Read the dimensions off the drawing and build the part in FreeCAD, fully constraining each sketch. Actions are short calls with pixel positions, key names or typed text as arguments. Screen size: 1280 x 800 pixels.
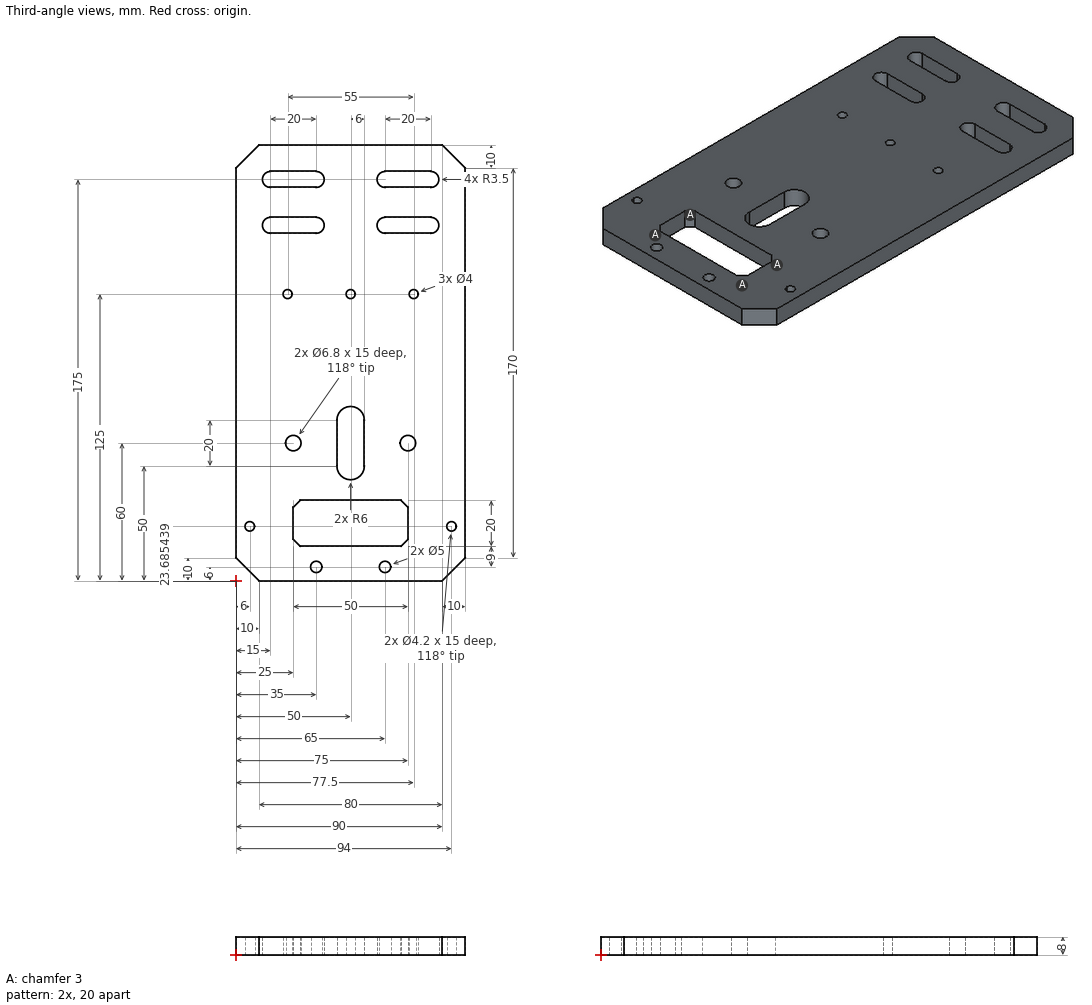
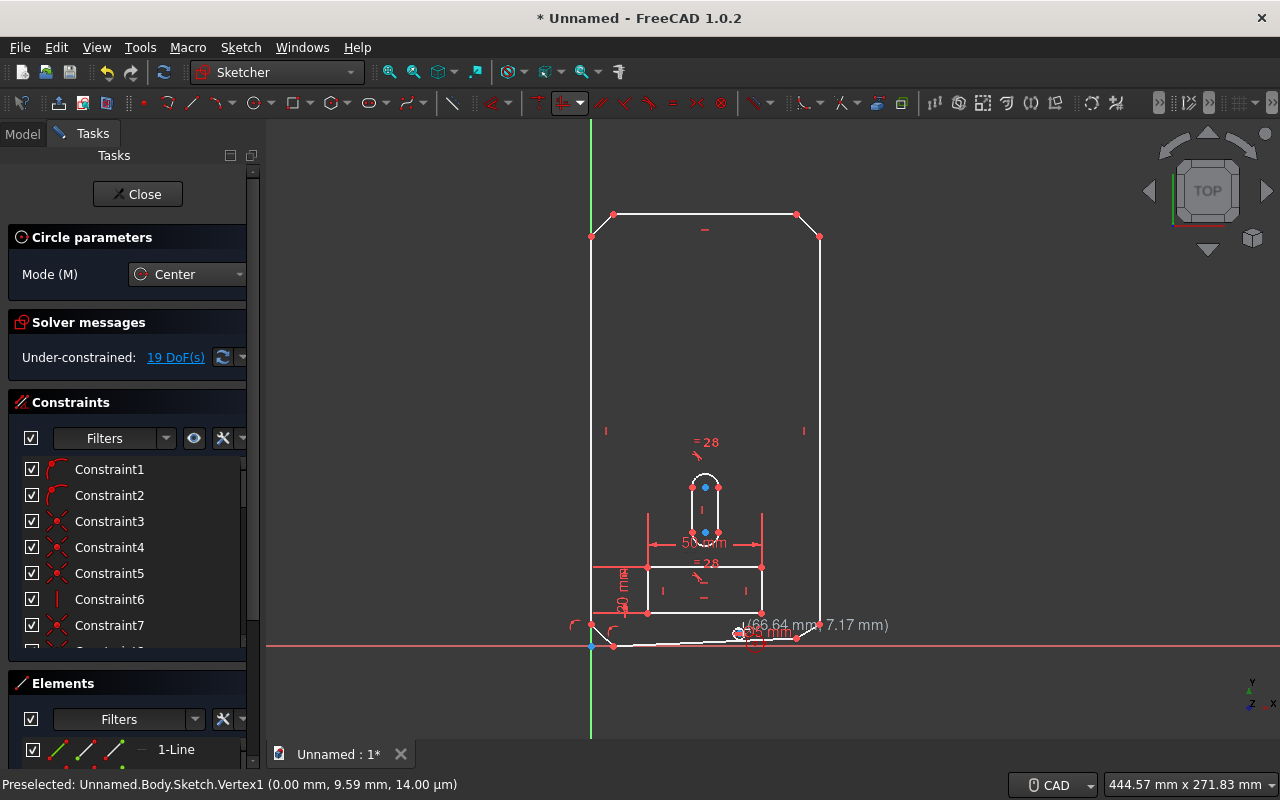
scroll(671, 633, up, 7)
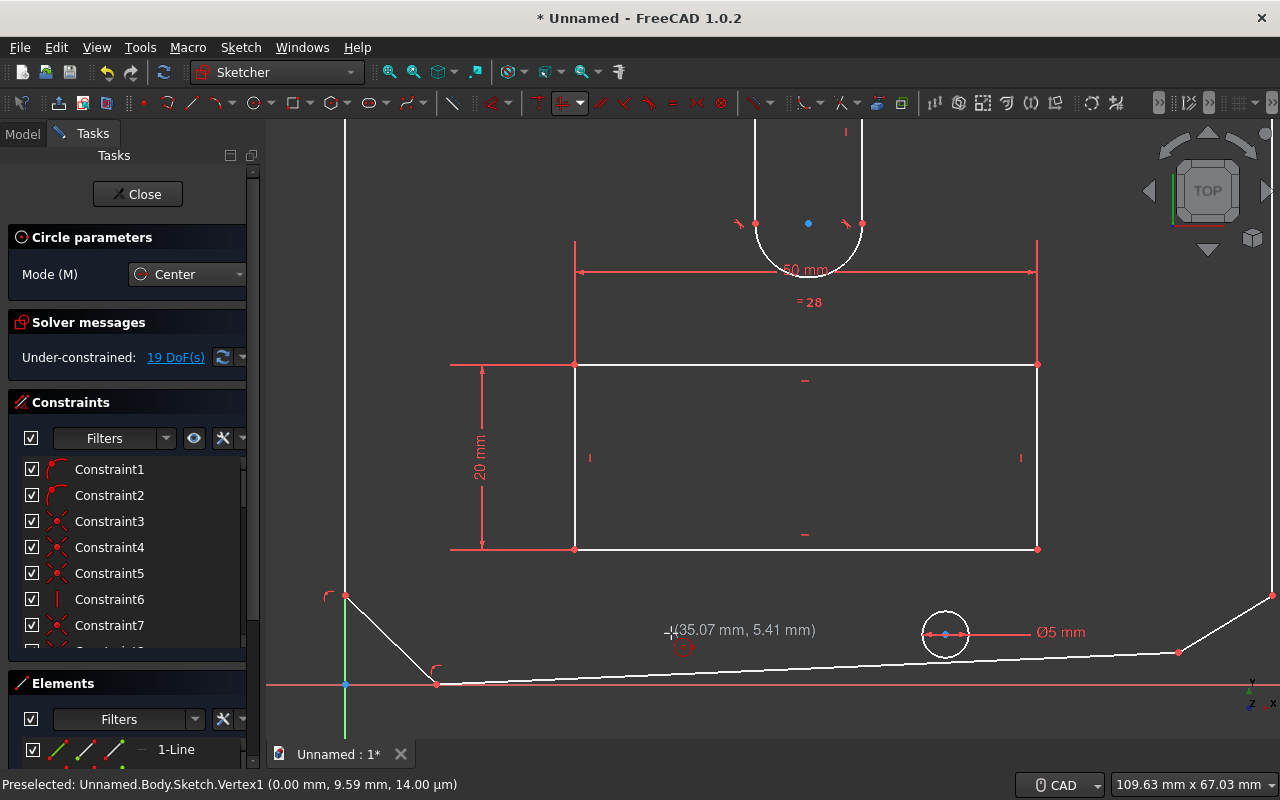
scroll(671, 633, down, 7)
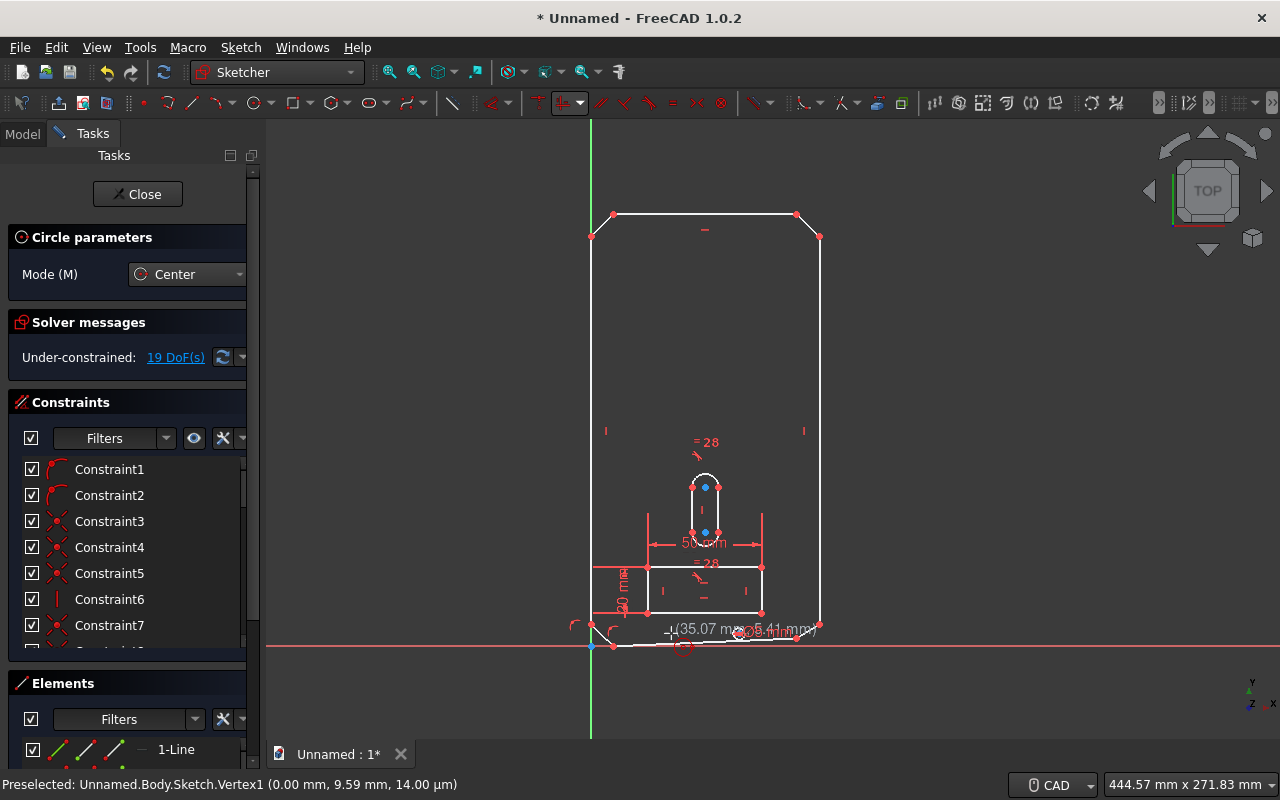
click(671, 633)
move(675, 629)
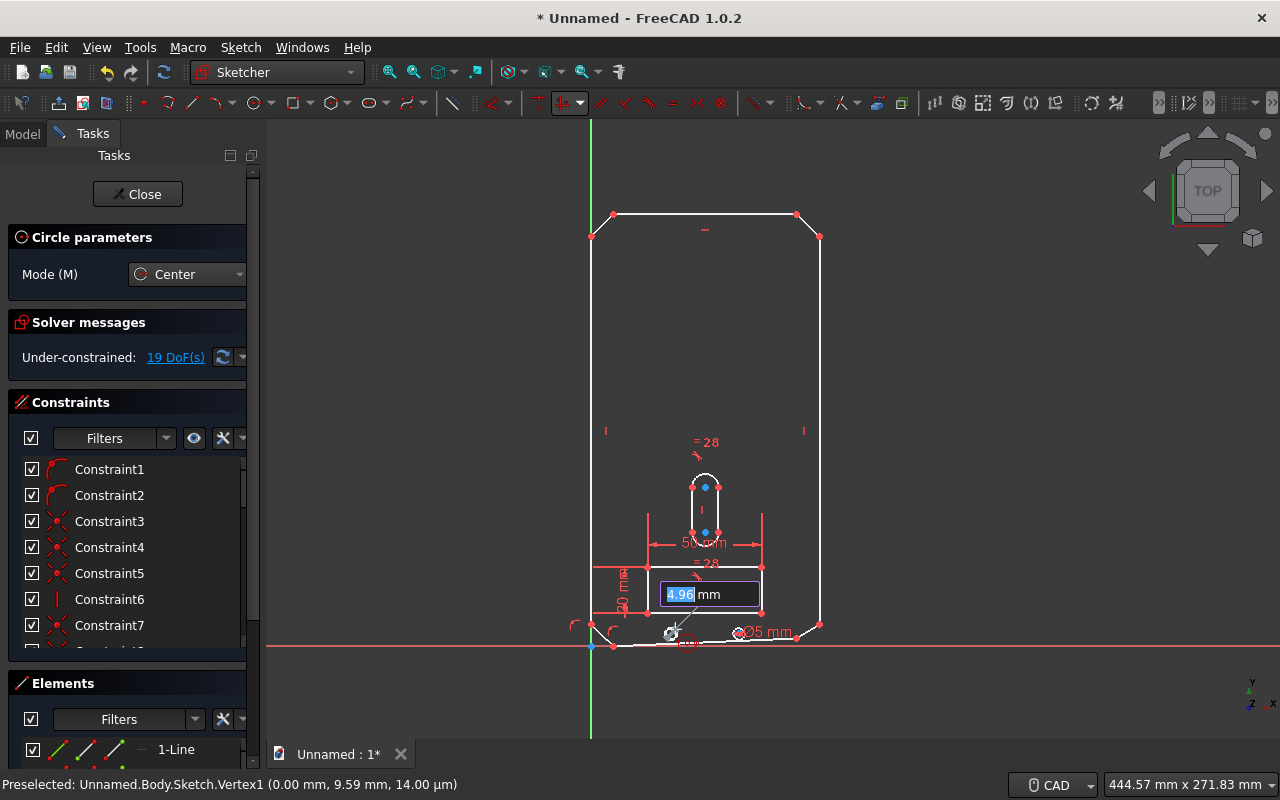
text(5)
key(Return)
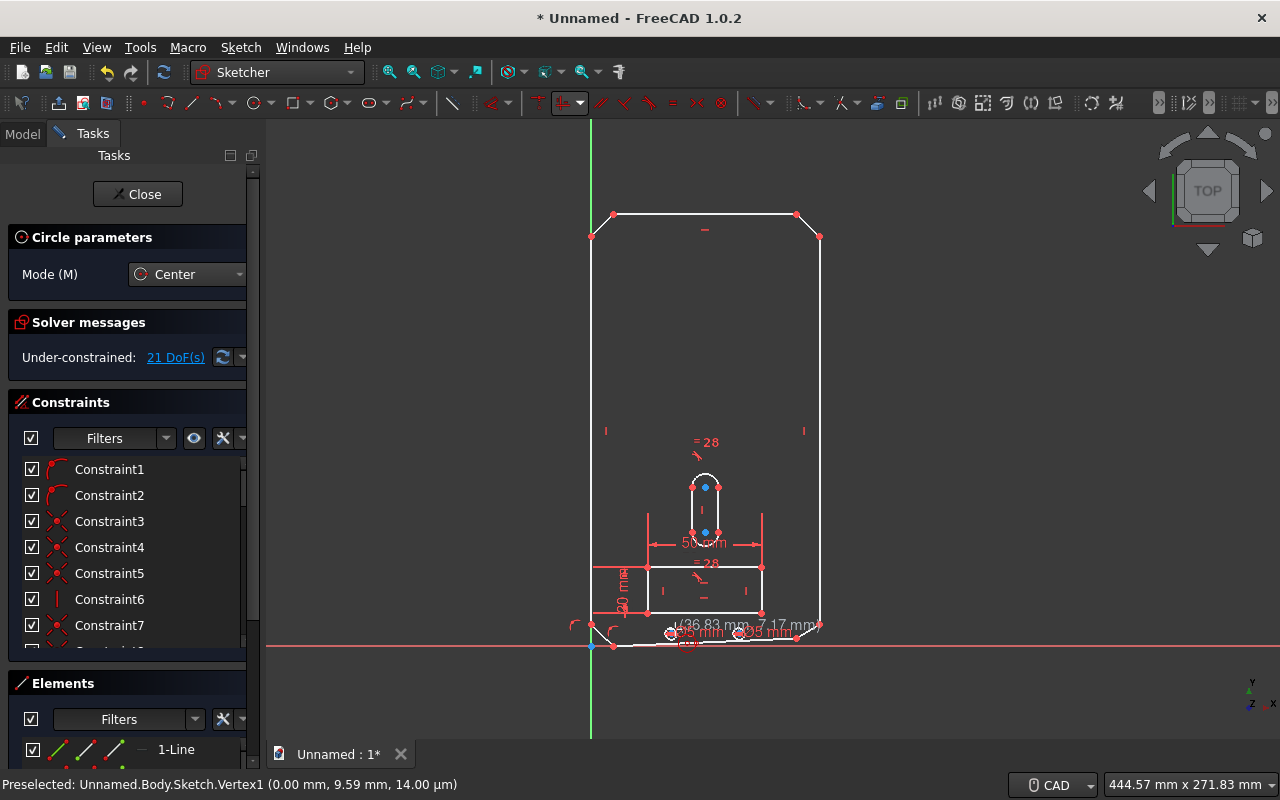
scroll(768, 361, up, 9)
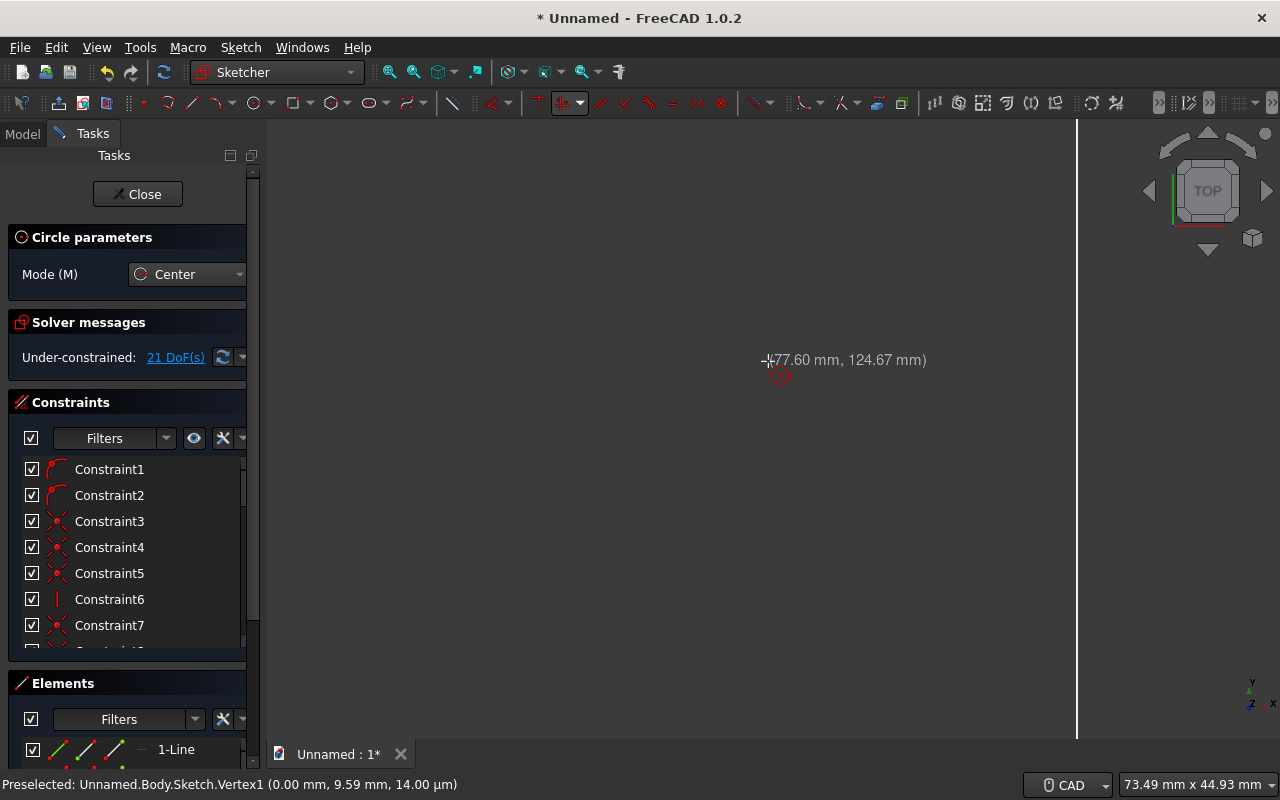
scroll(768, 361, down, 9)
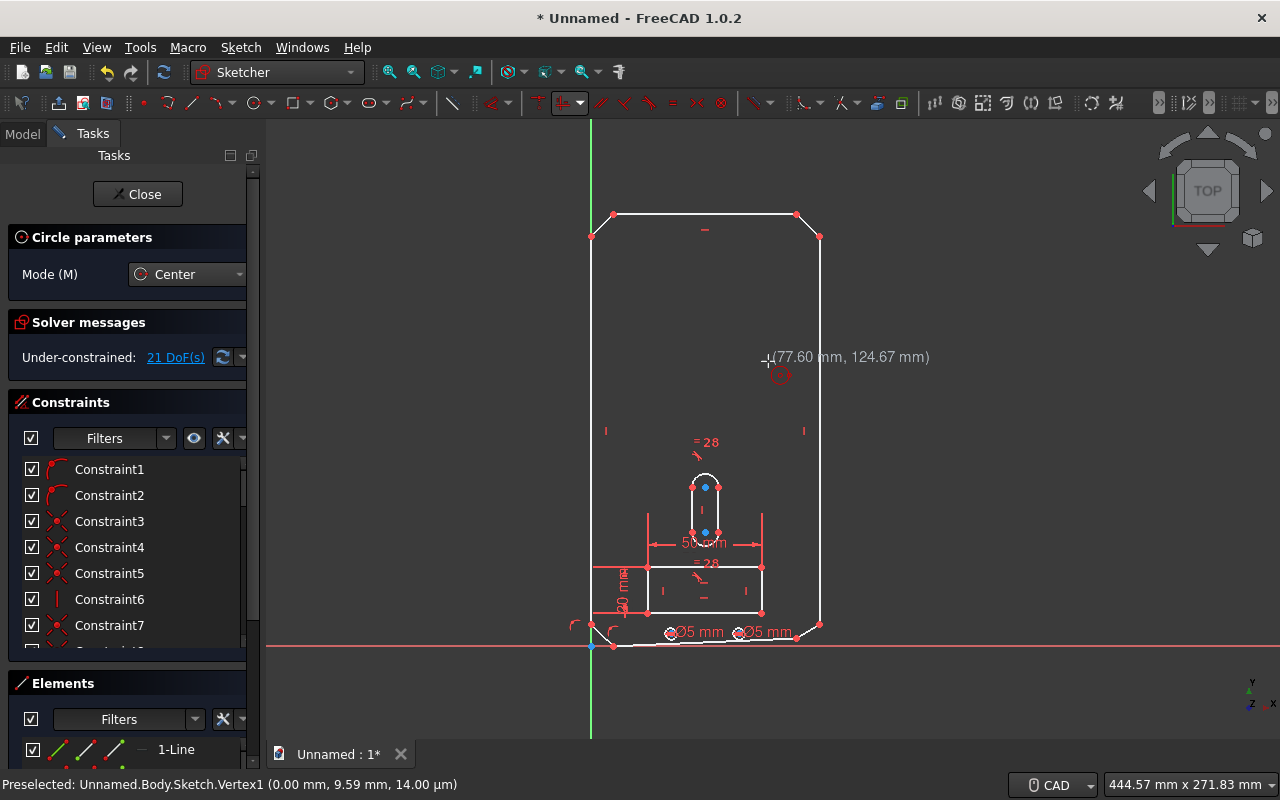
click(768, 361)
move(771, 358)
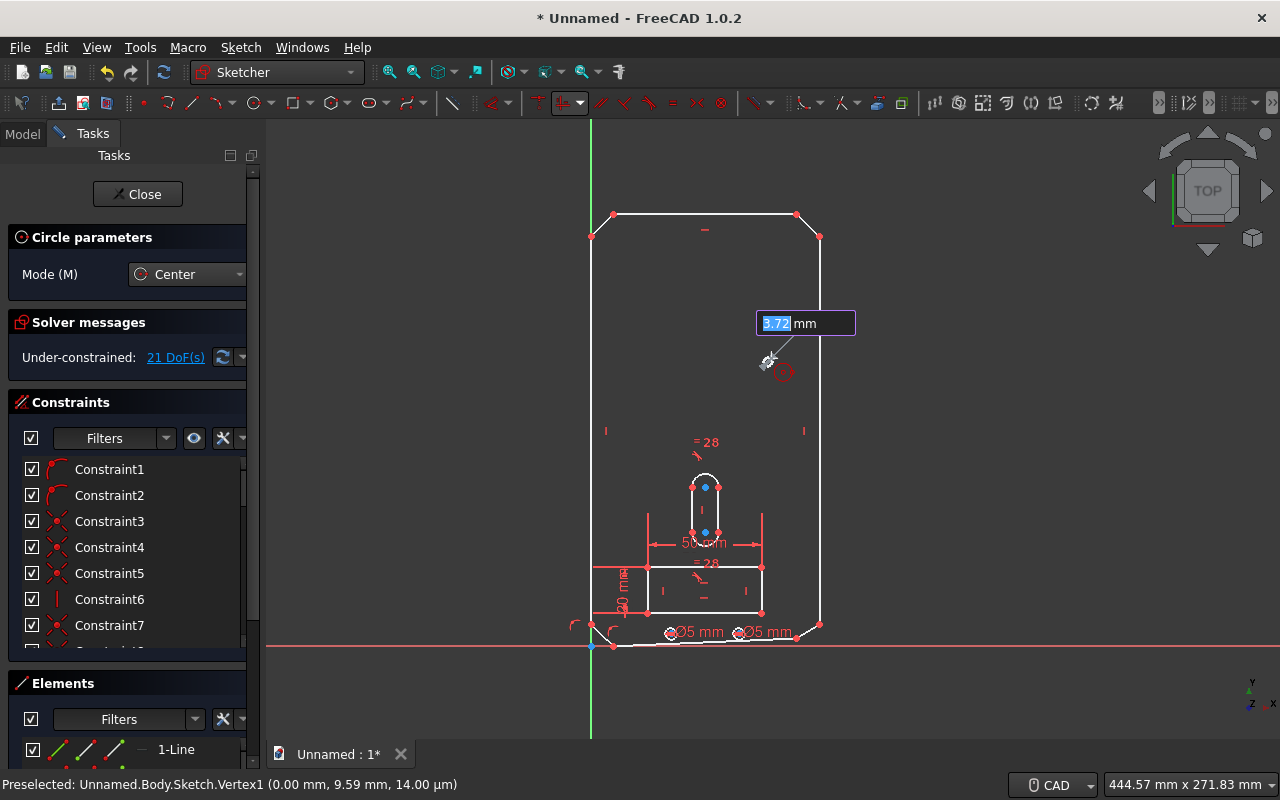
text(4)
key(Return)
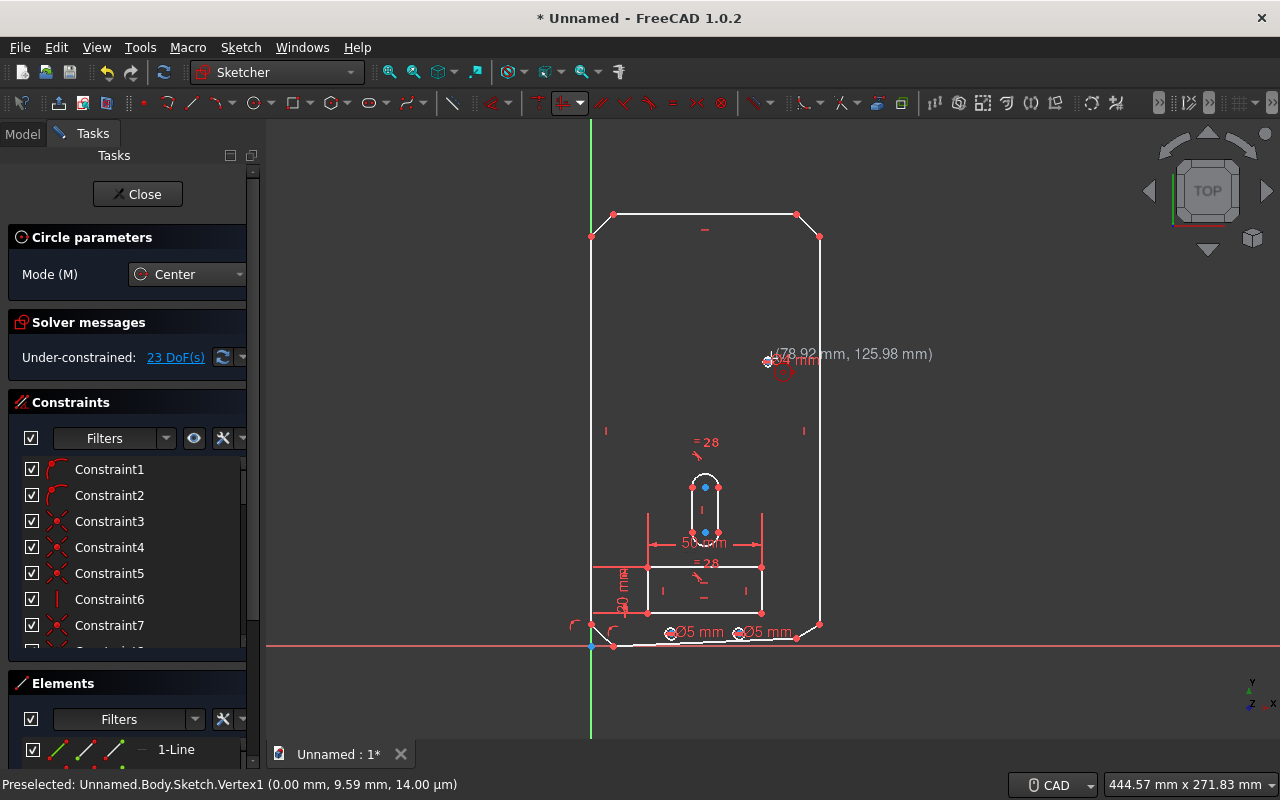
scroll(705, 361, up, 9)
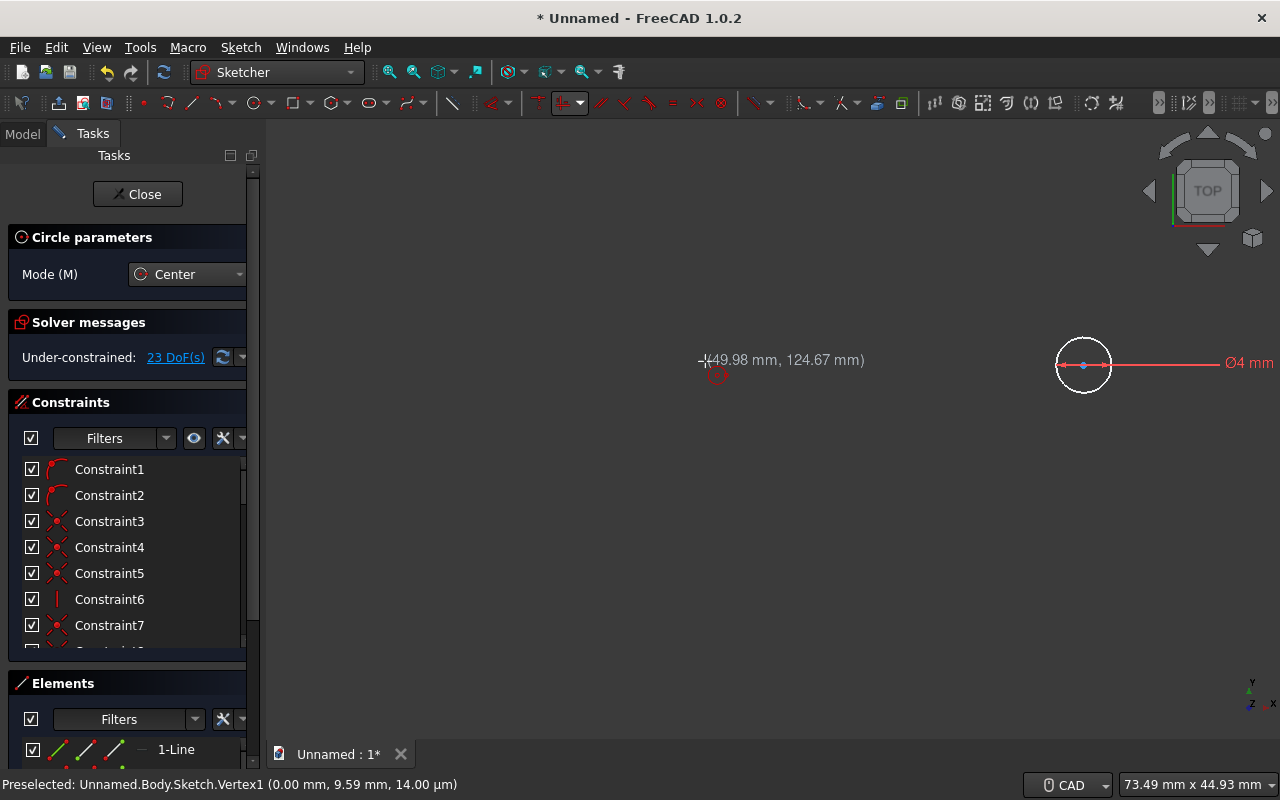
scroll(705, 361, down, 9)